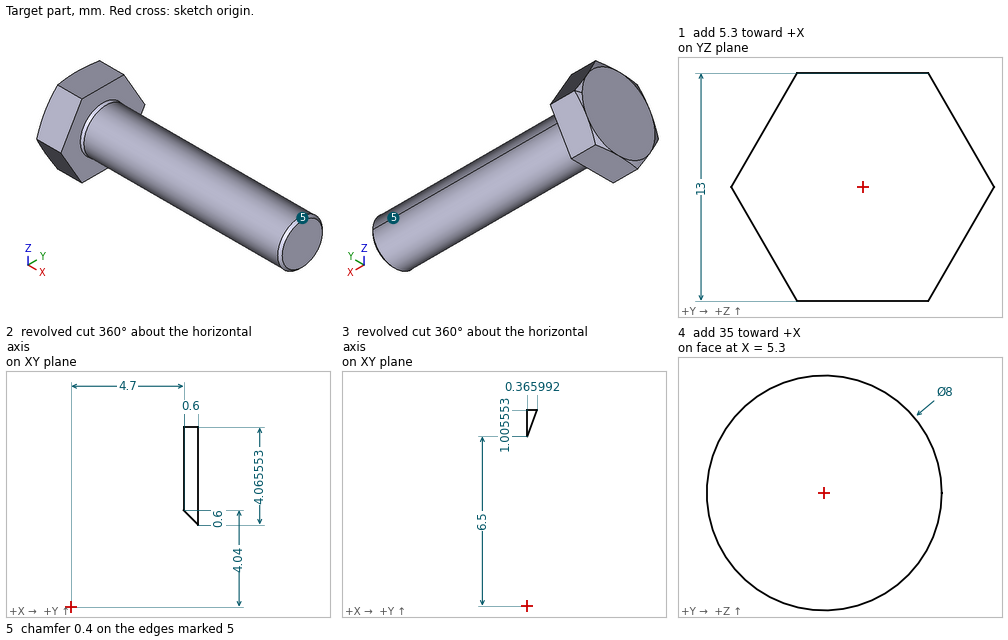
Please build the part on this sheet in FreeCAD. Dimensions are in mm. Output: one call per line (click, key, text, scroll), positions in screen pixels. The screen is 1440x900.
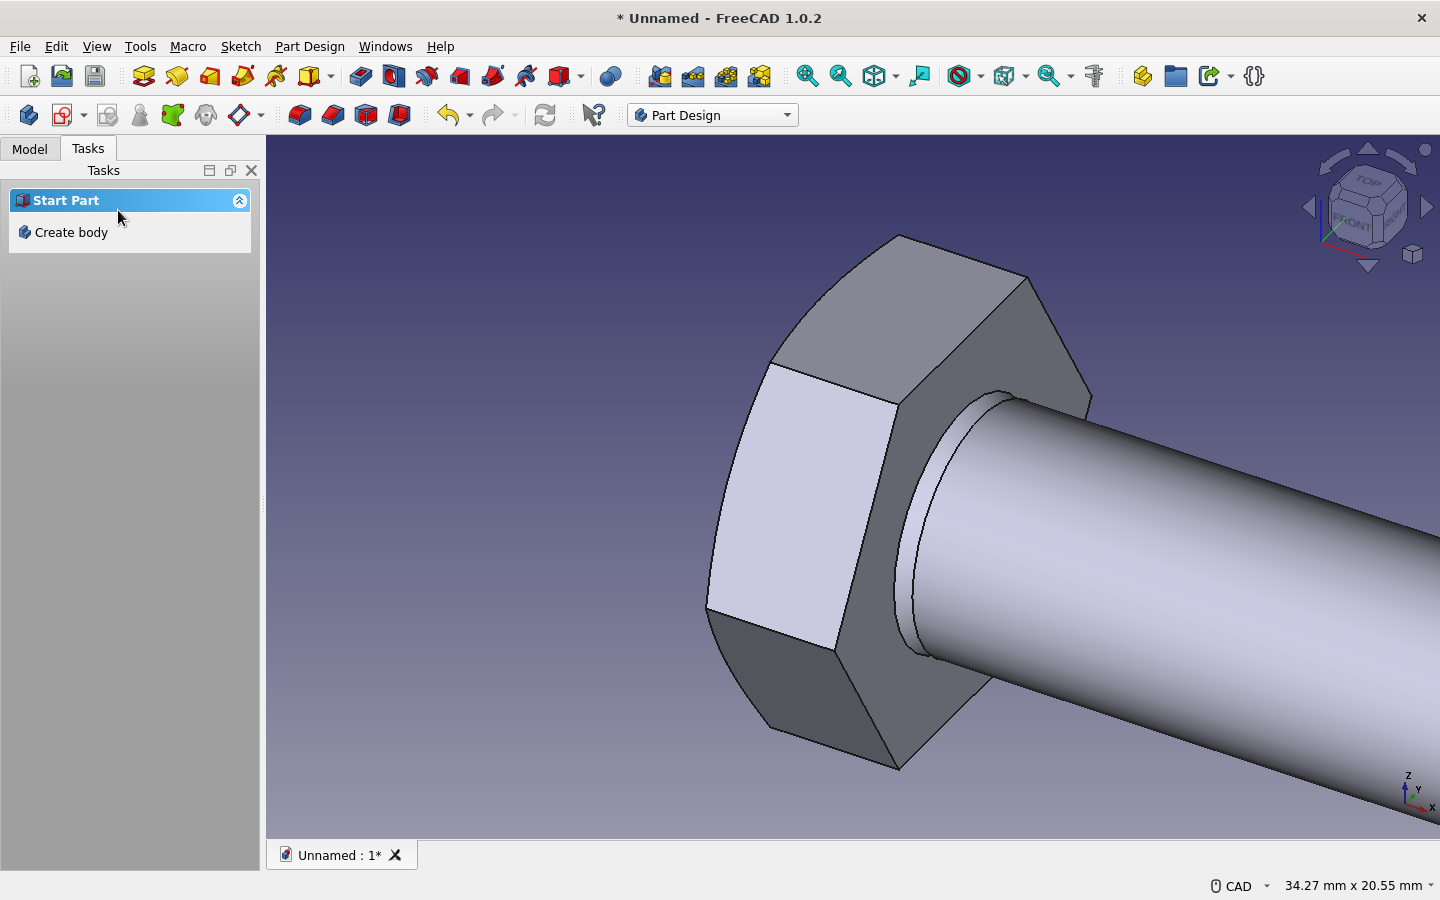
key(v)
key(f)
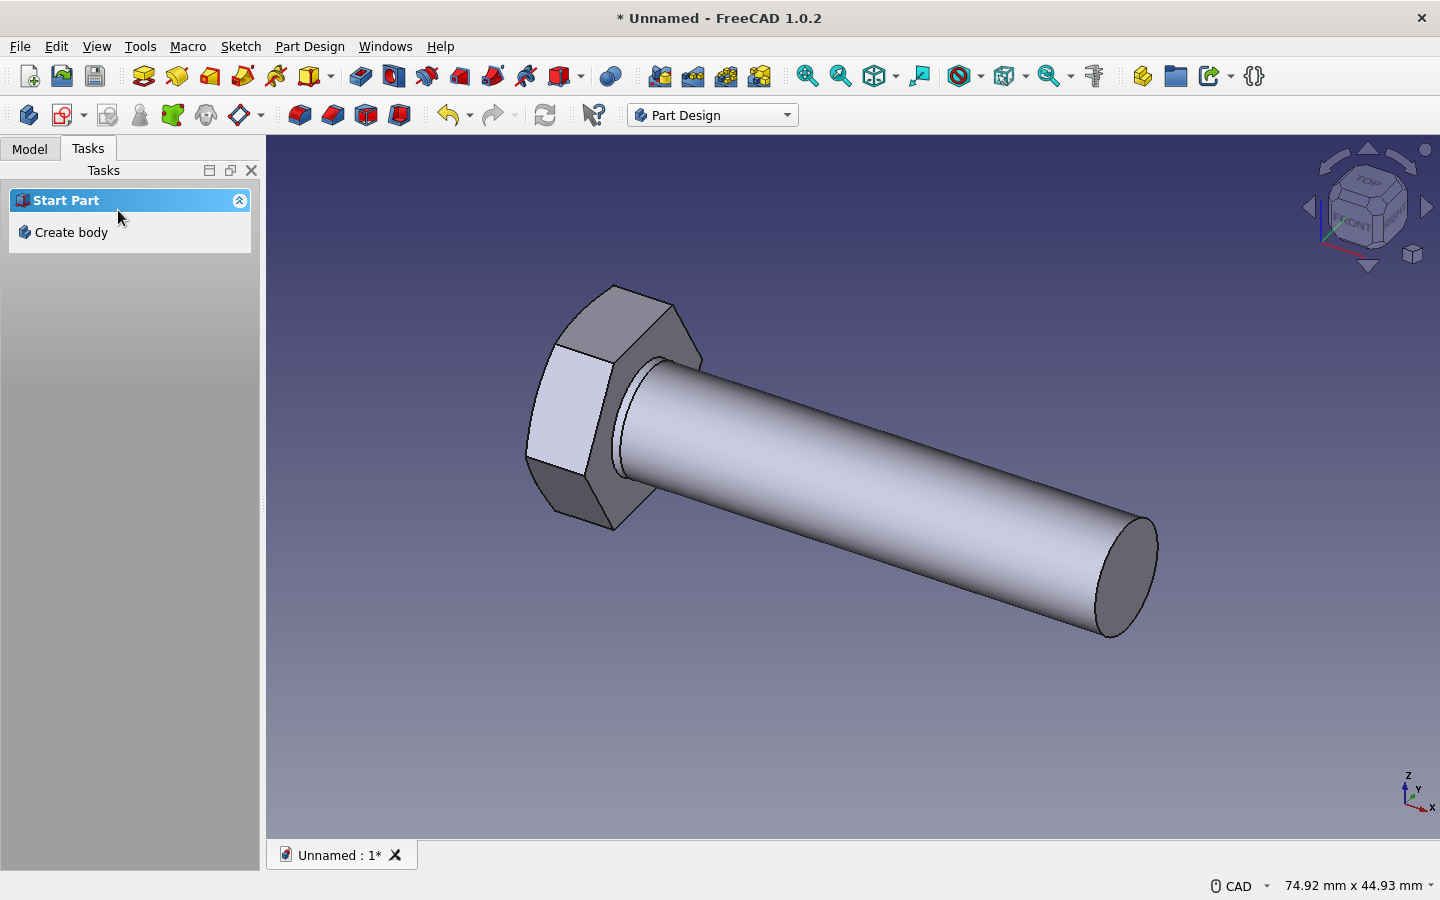
click(1095, 608)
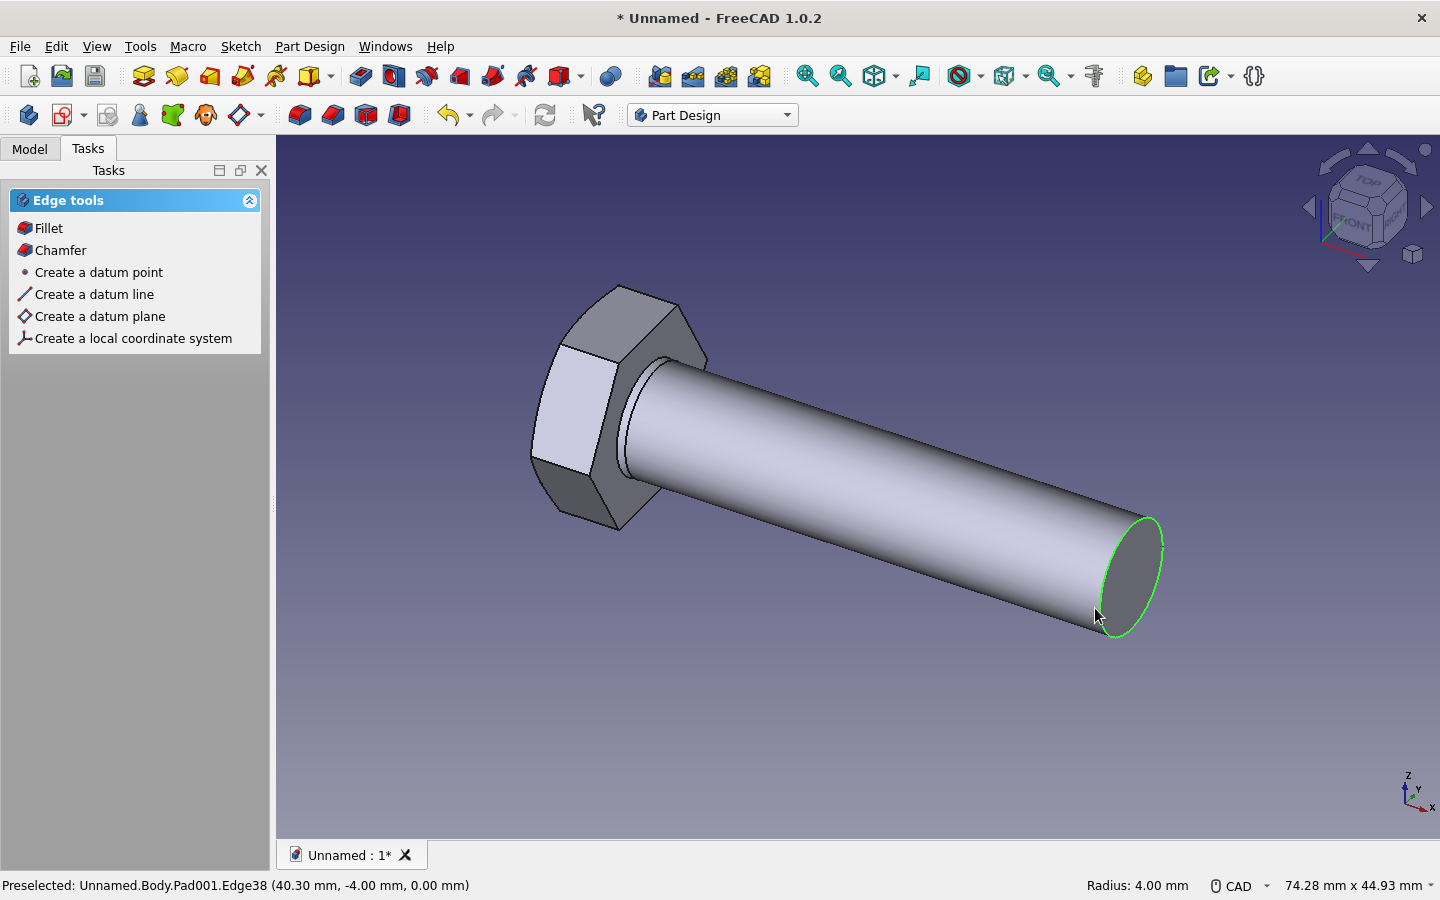
click(333, 116)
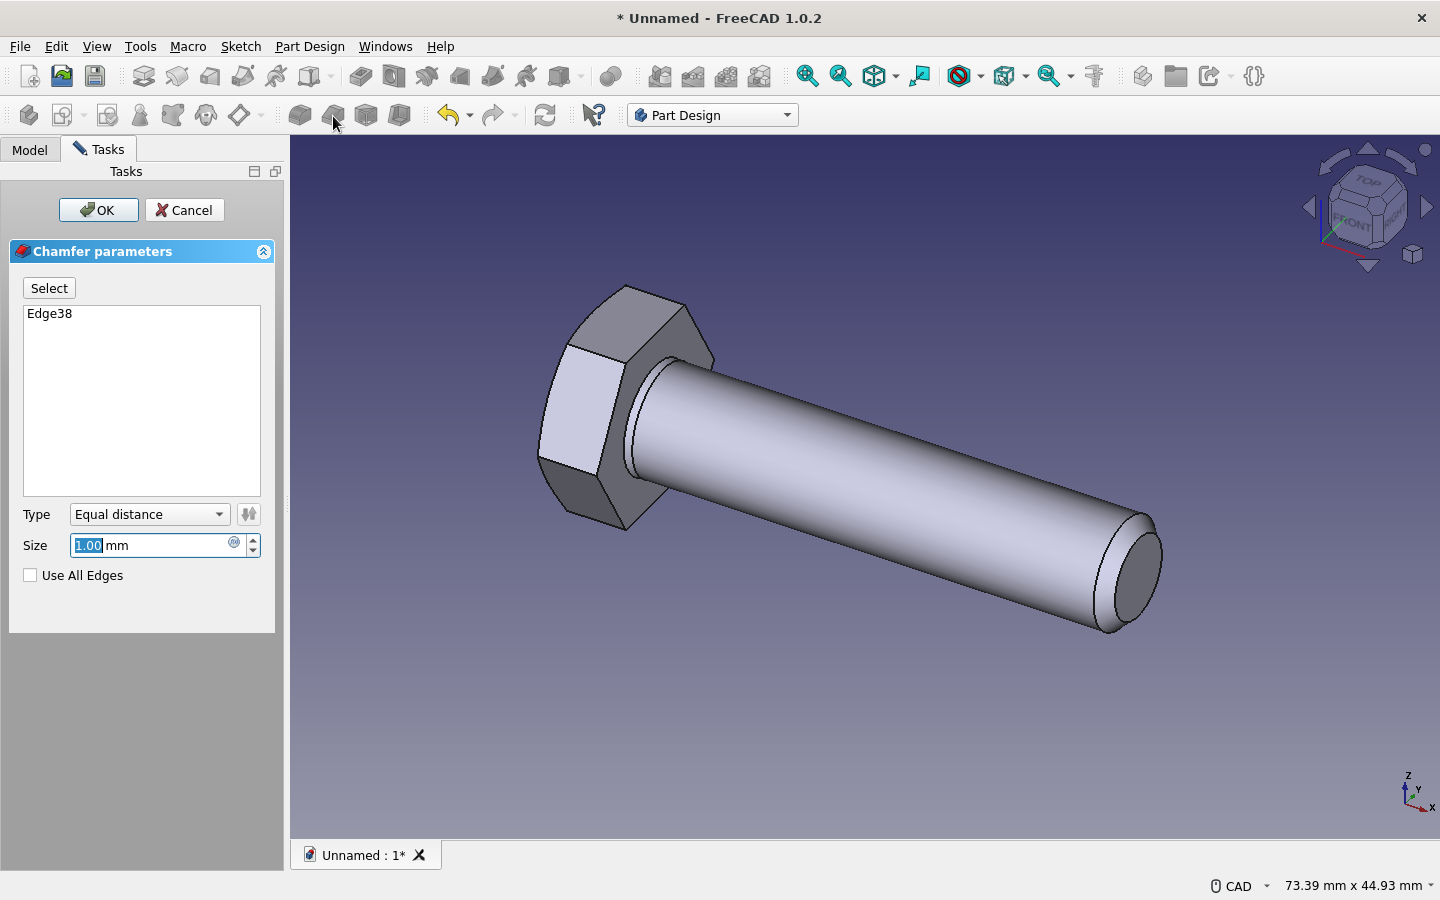
text(0.4)
key(Tab)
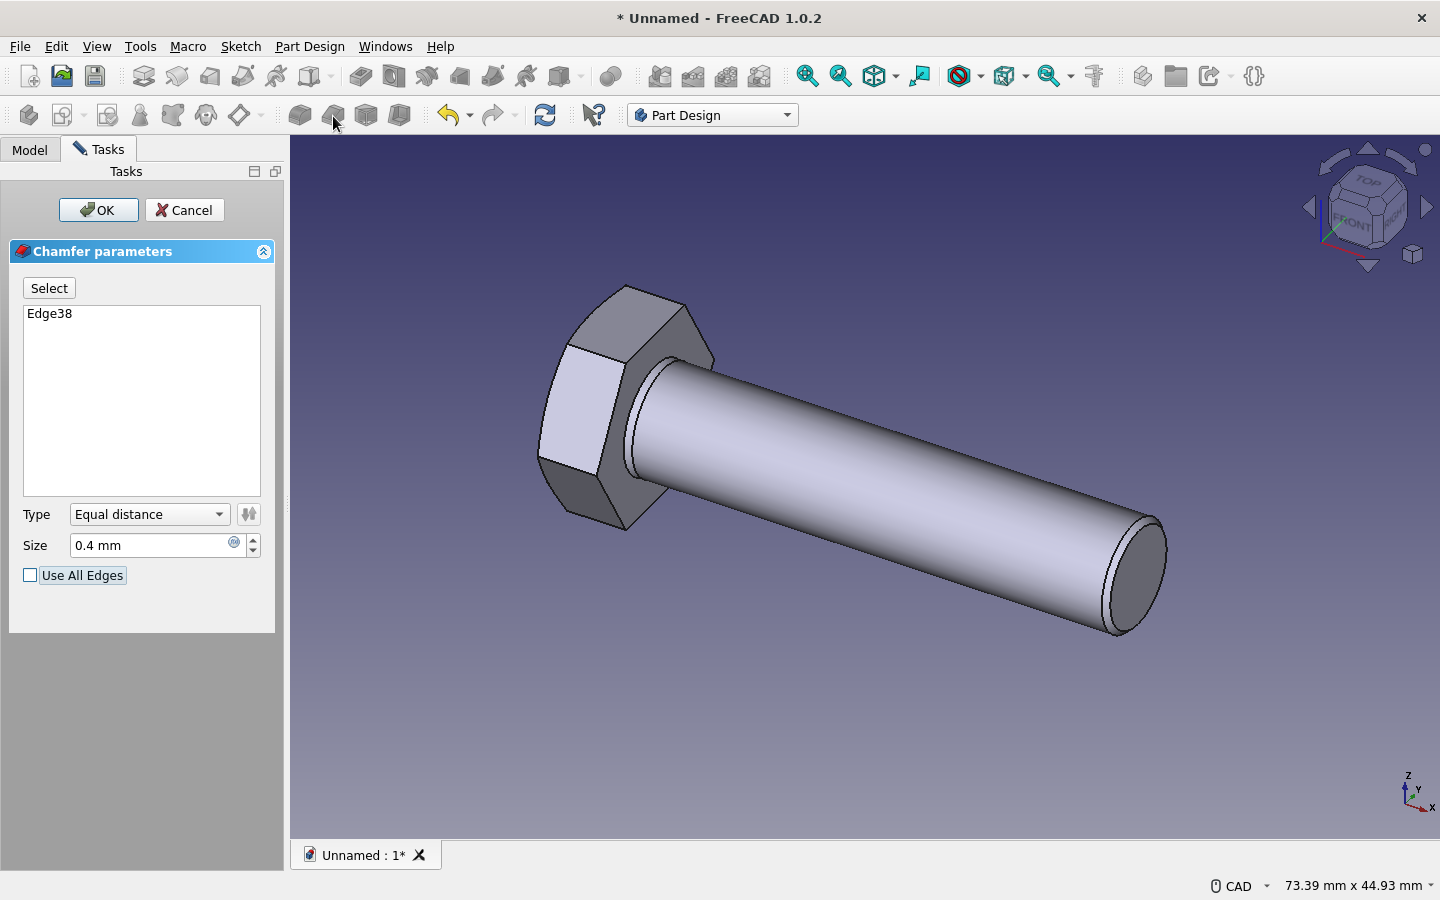
click(99, 210)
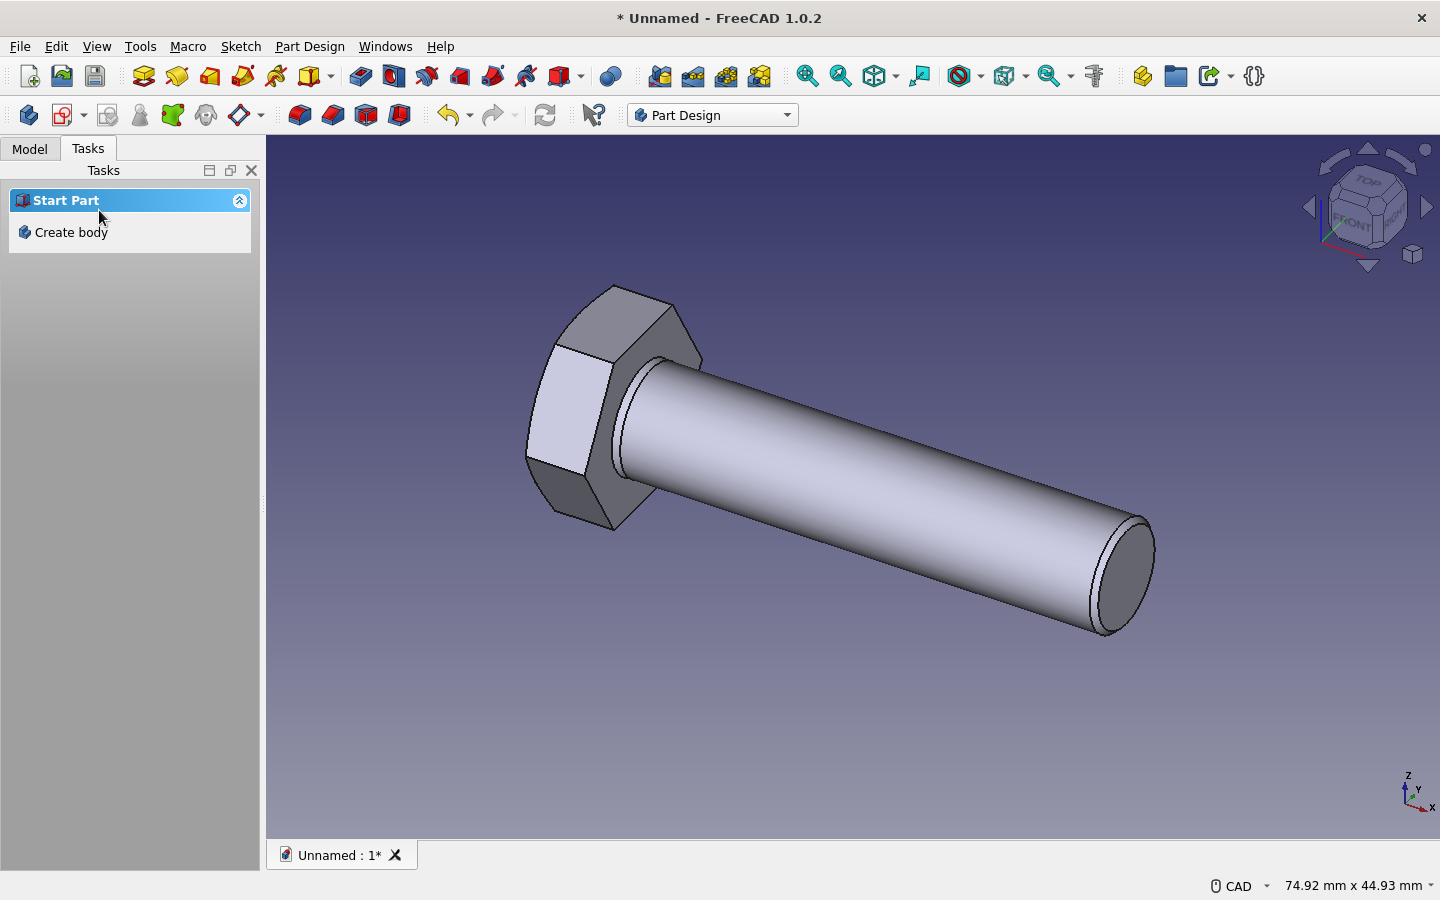
key(0)